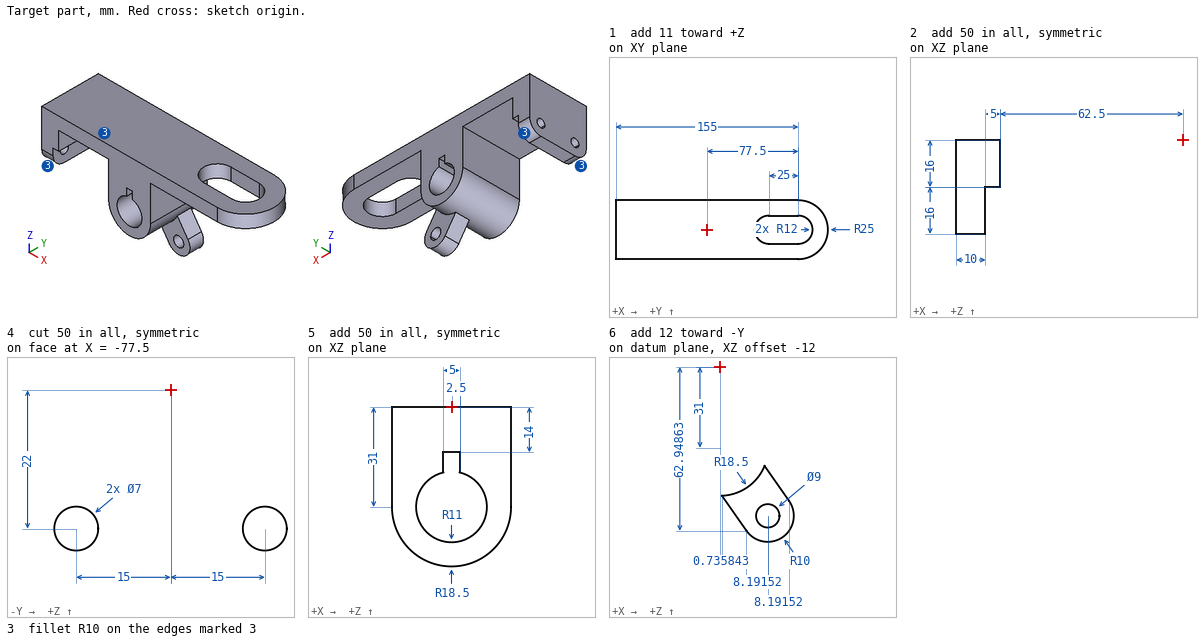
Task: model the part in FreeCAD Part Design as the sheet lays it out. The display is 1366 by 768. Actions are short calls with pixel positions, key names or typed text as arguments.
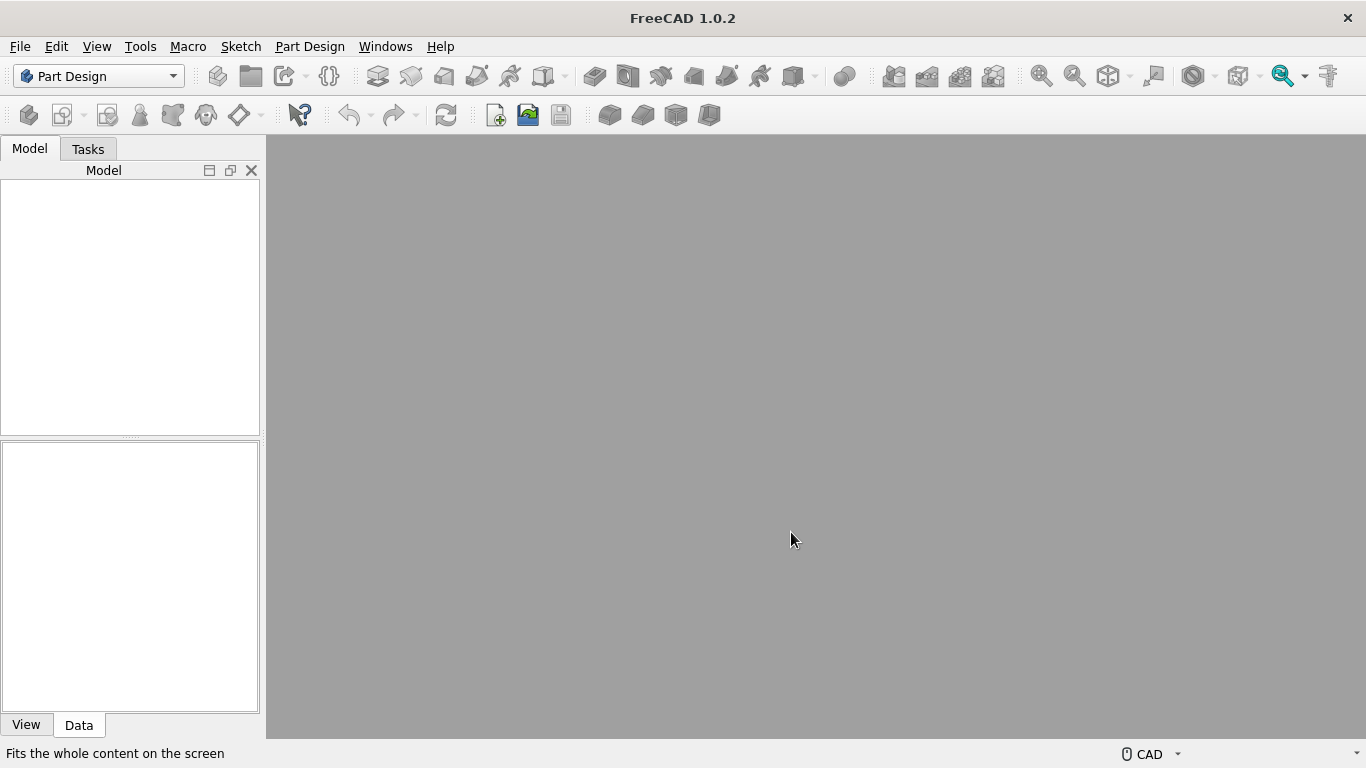
key(ctrl+n)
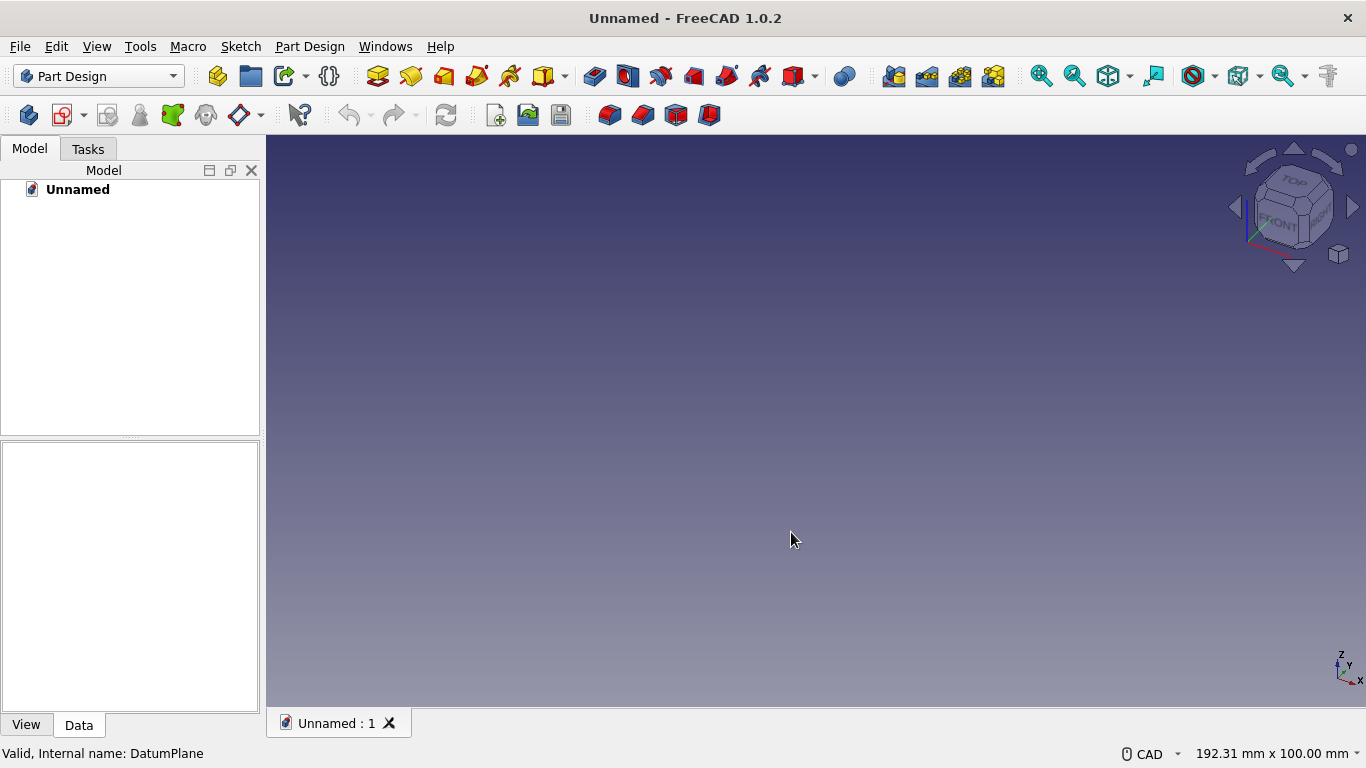
click(62, 116)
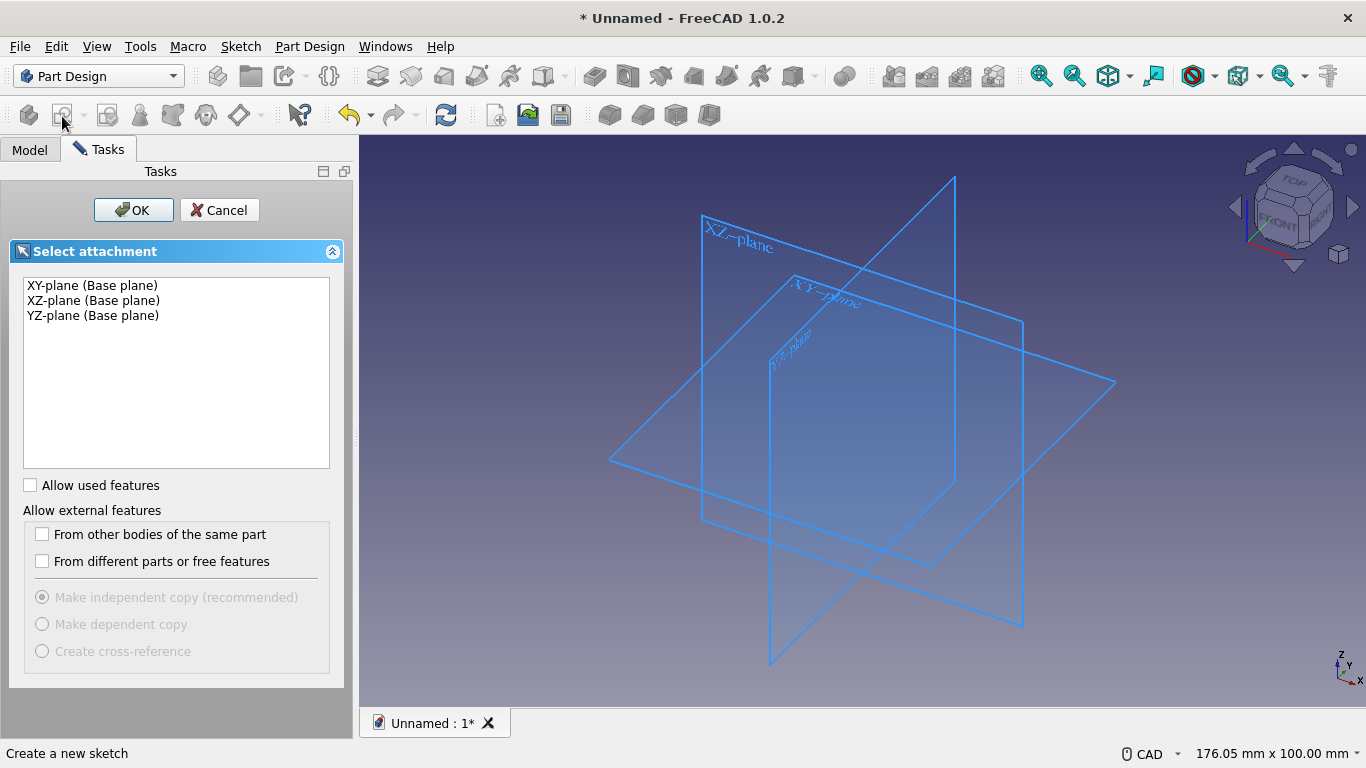
click(84, 286)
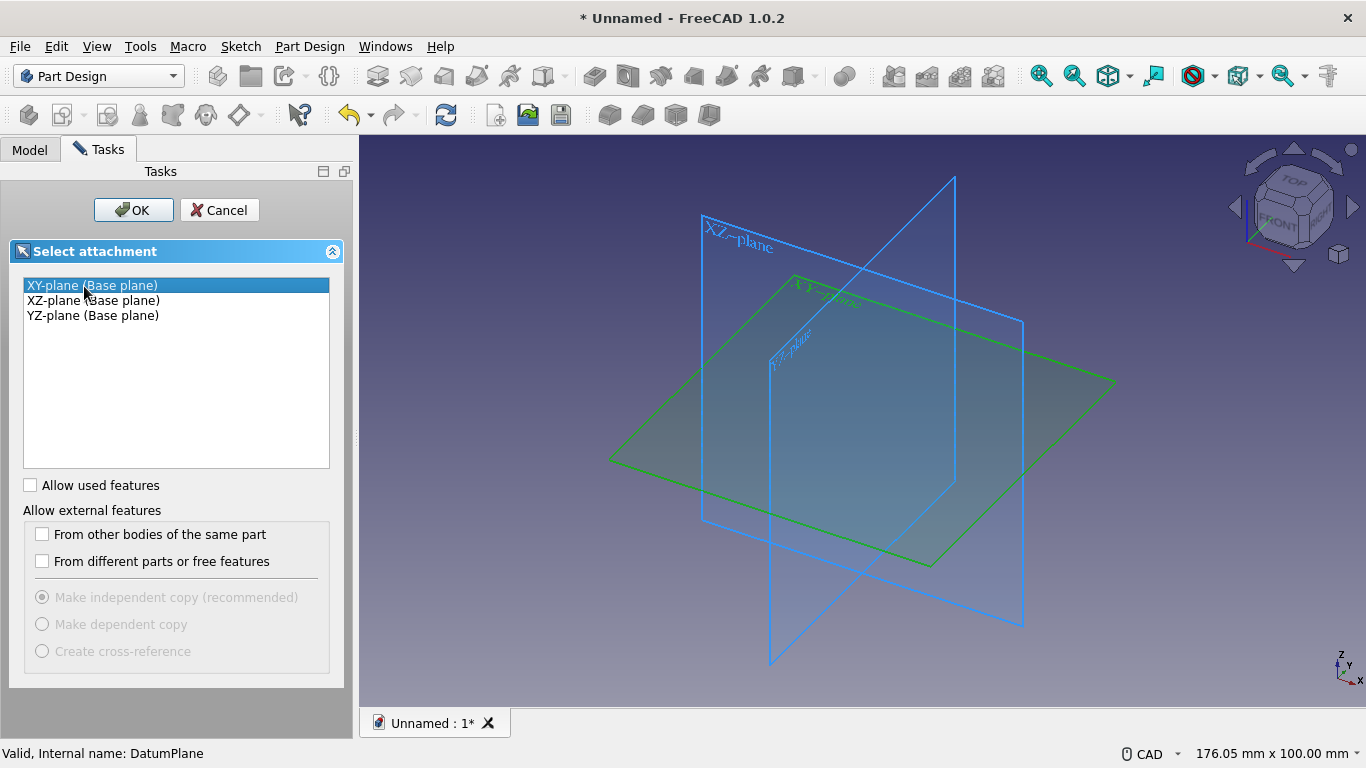
click(134, 210)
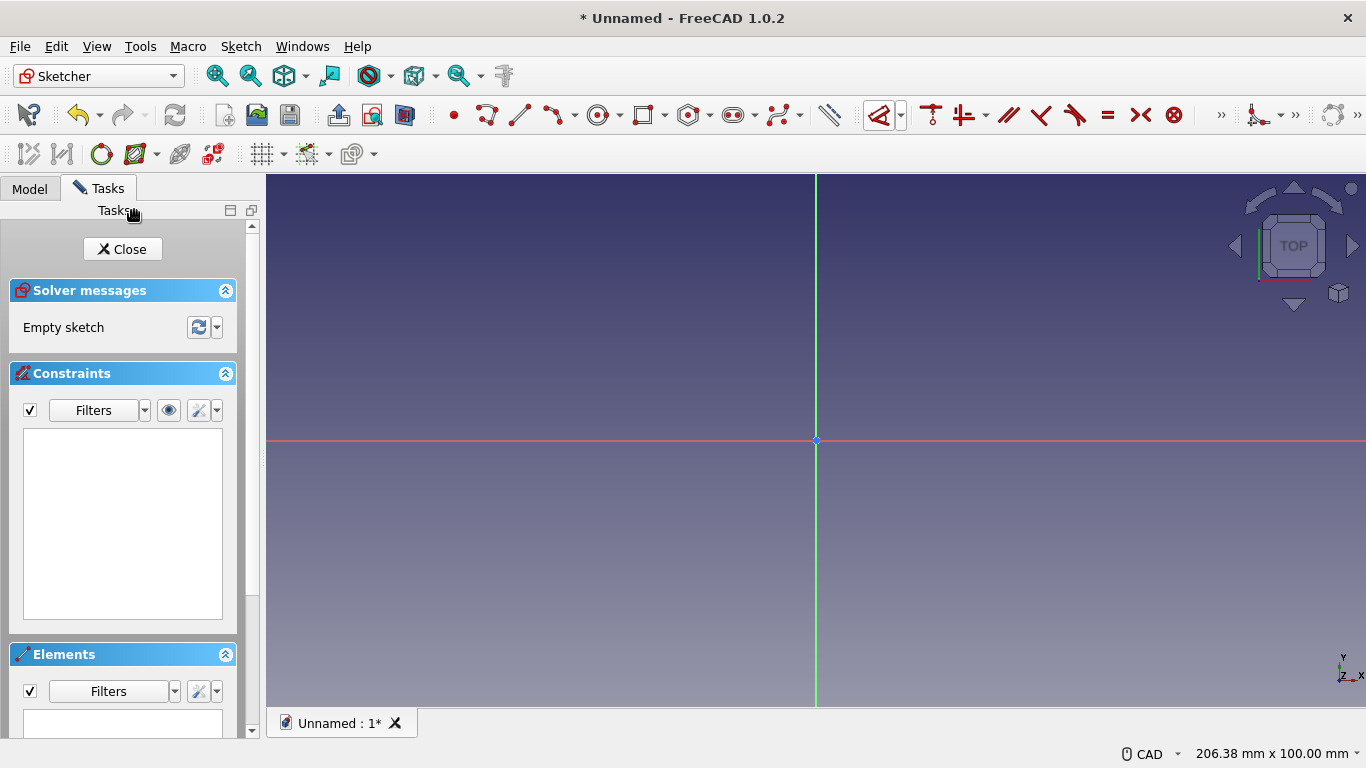
scroll(473, 440, down, 2)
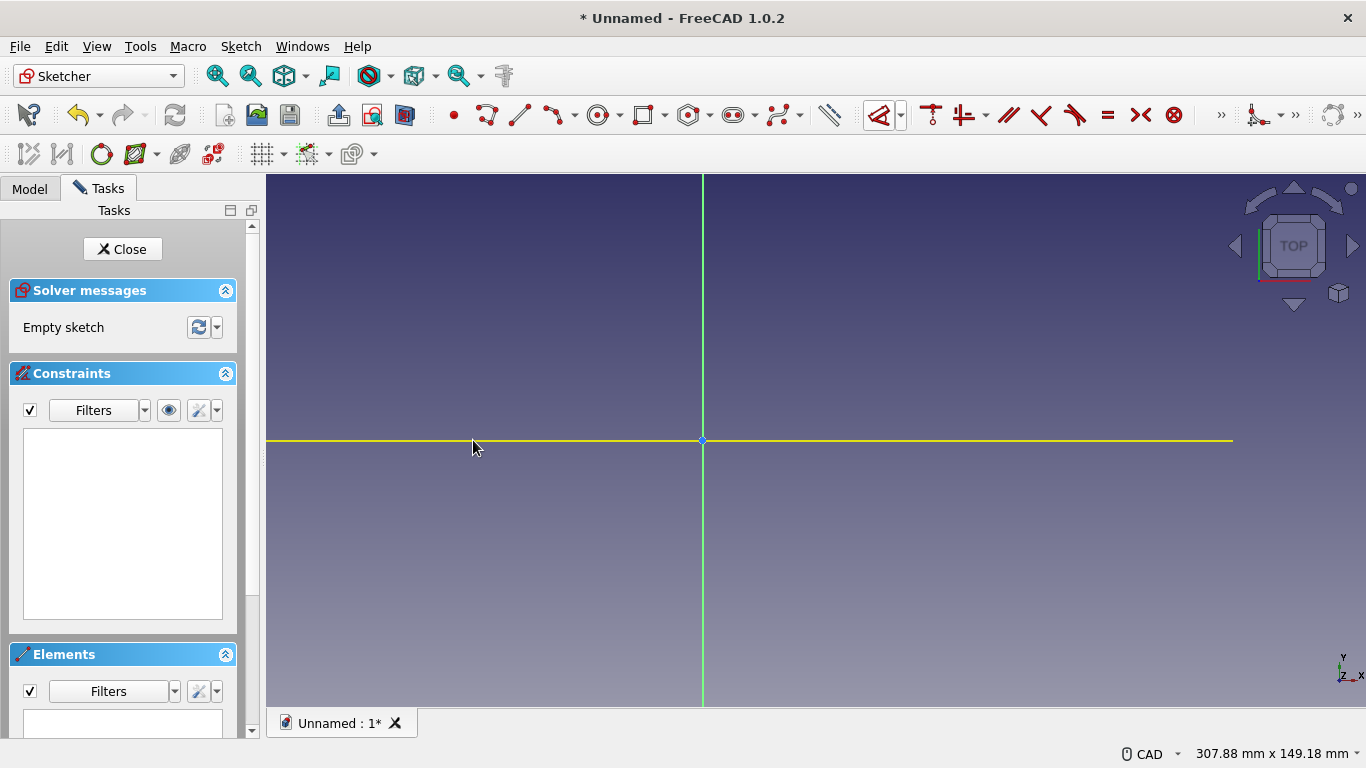
click(487, 116)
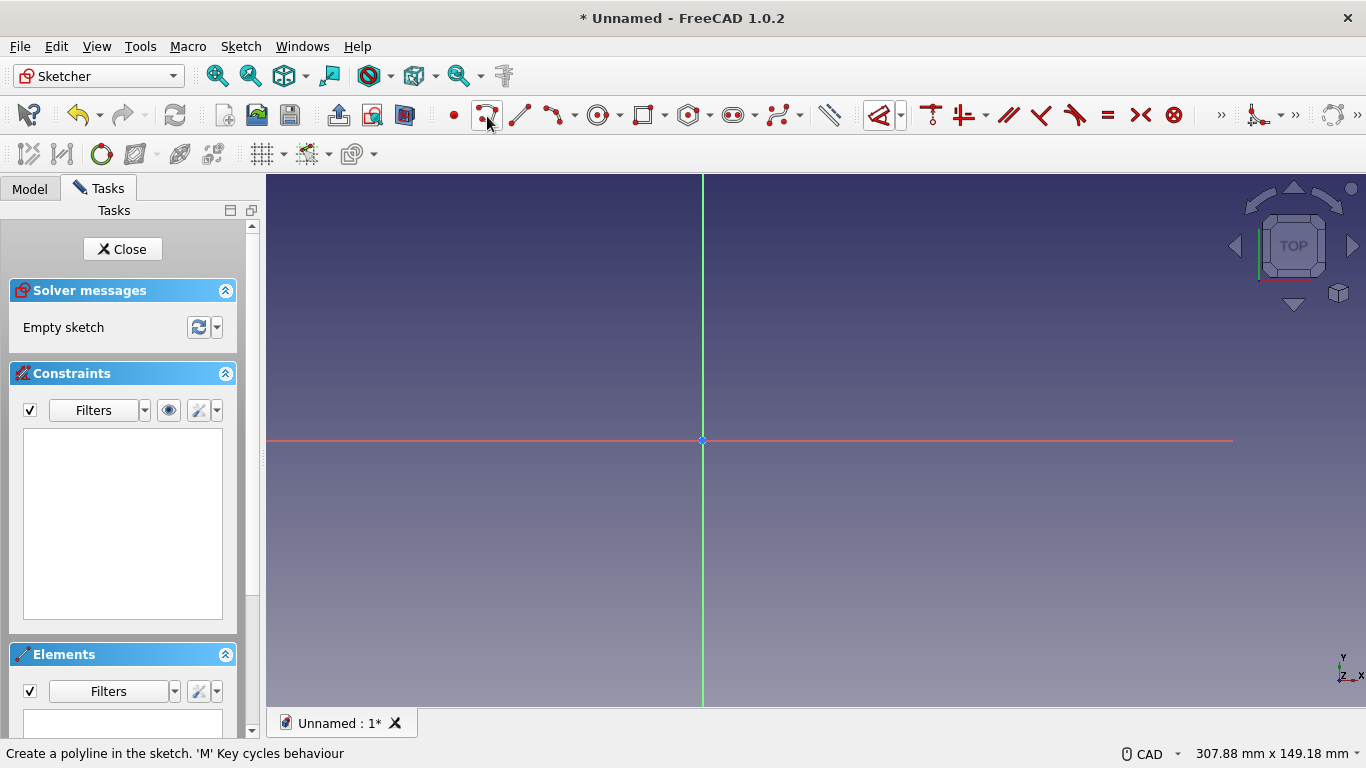
click(980, 351)
click(426, 351)
click(426, 530)
click(980, 530)
right_click(980, 530)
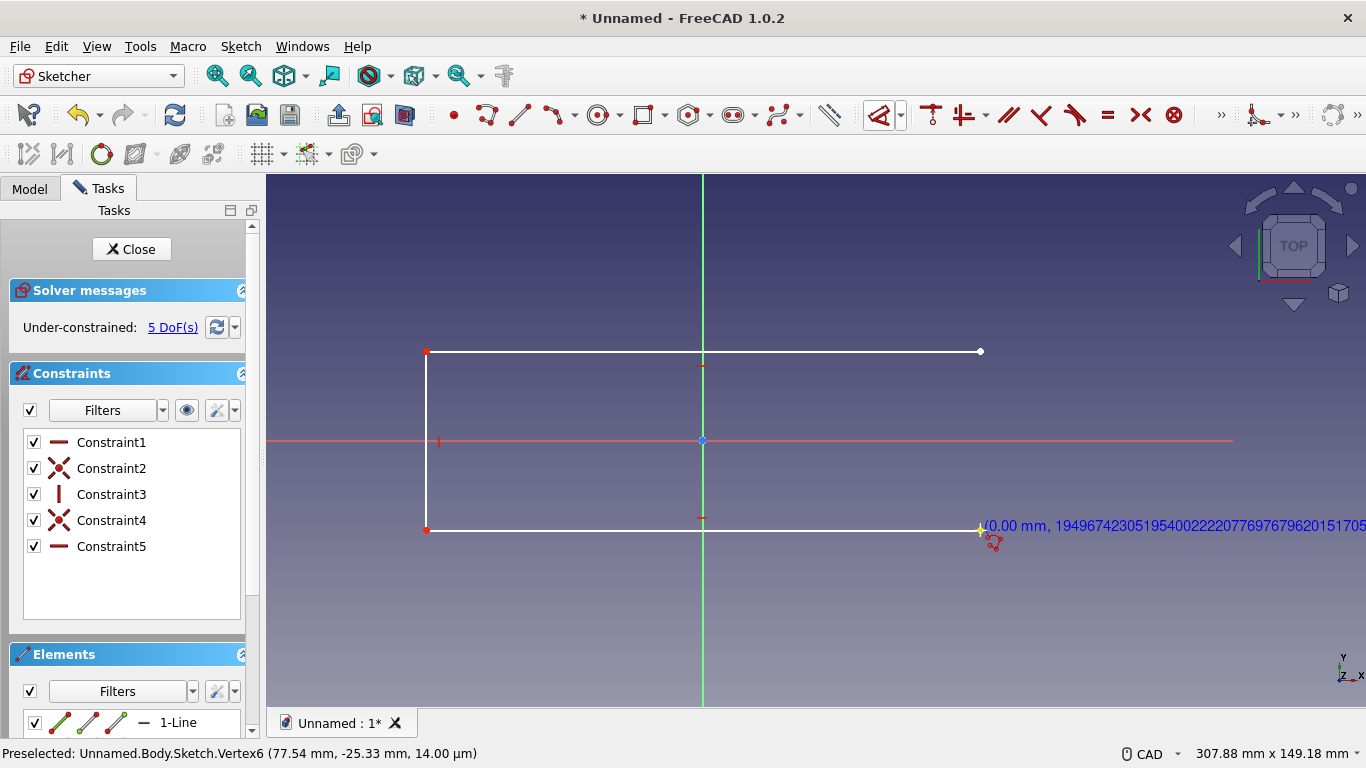
key(g)
key(3)
key(a)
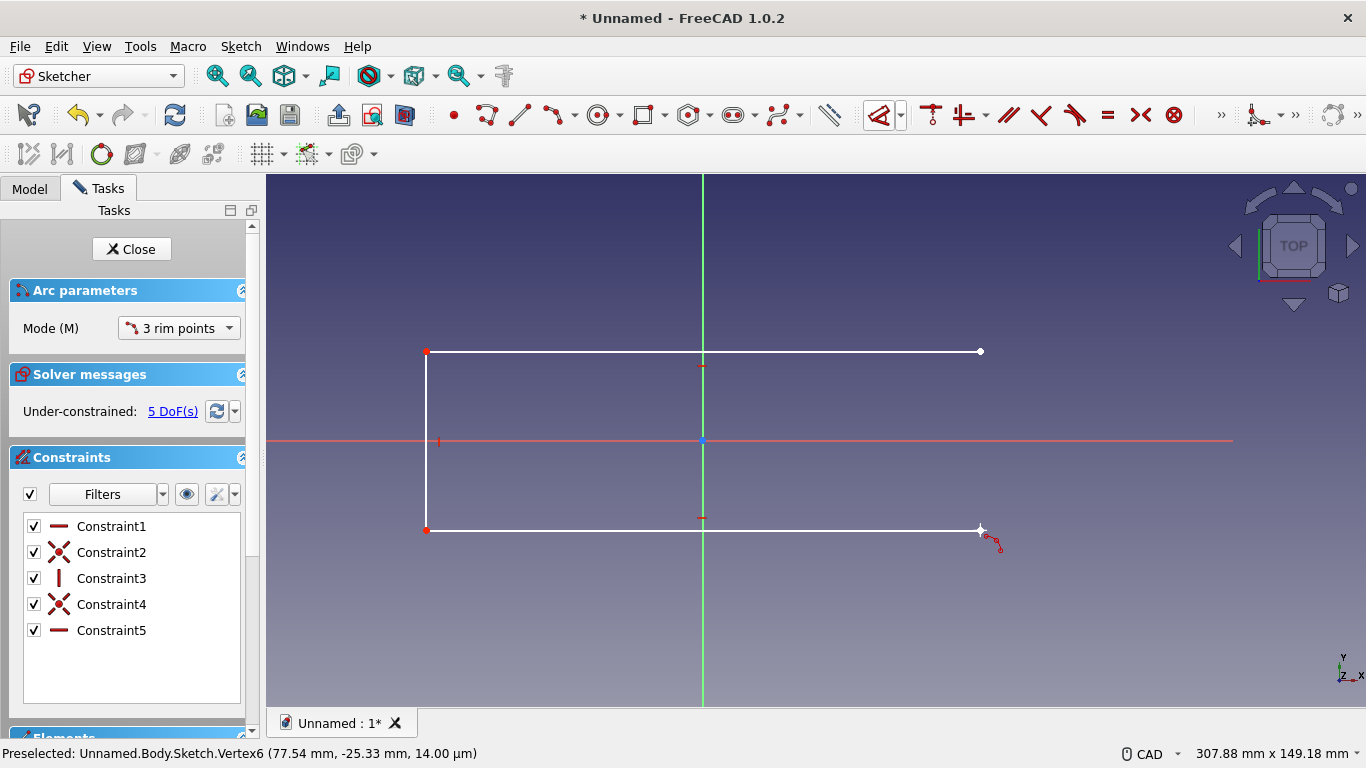
click(980, 531)
click(980, 352)
click(1065, 468)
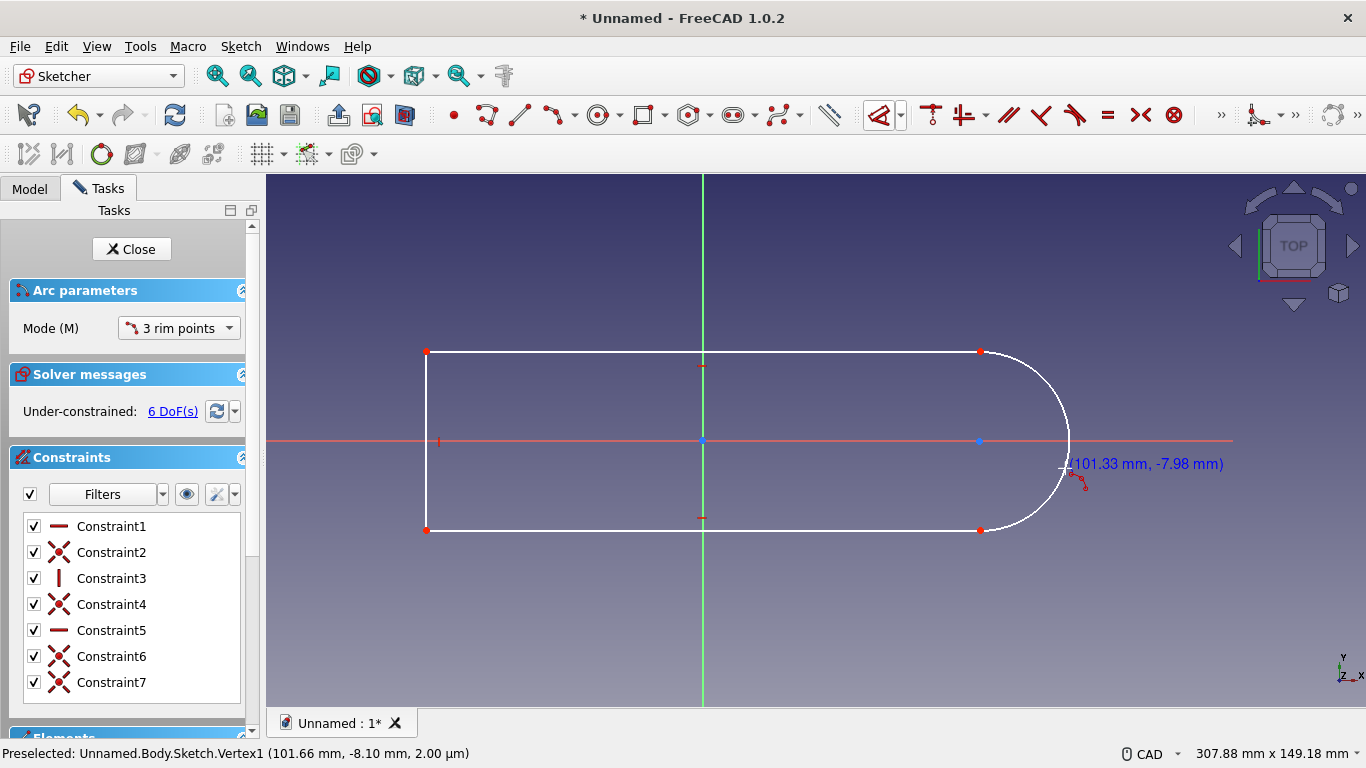
click(732, 116)